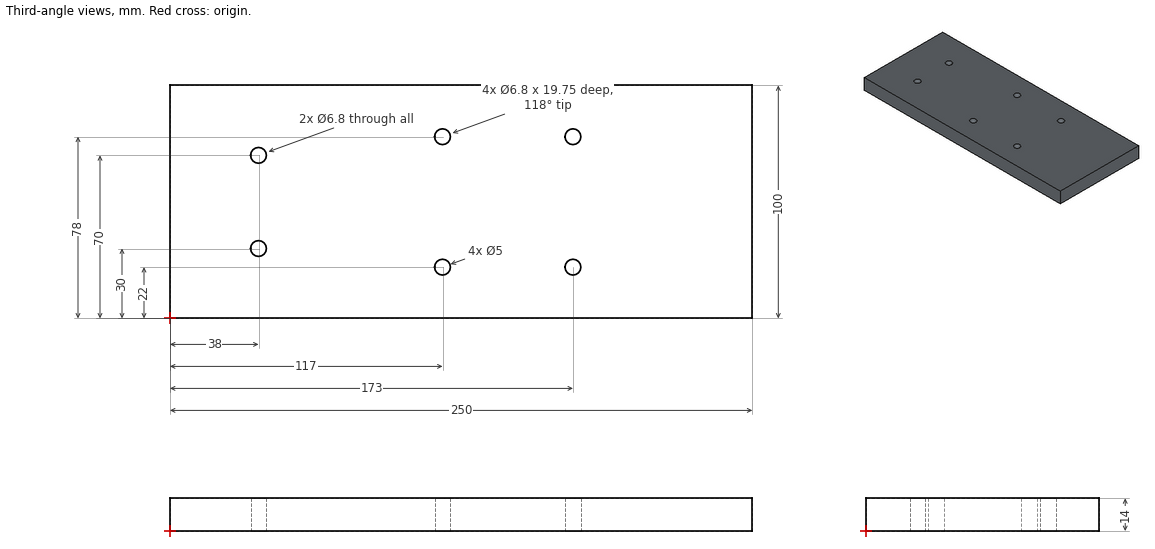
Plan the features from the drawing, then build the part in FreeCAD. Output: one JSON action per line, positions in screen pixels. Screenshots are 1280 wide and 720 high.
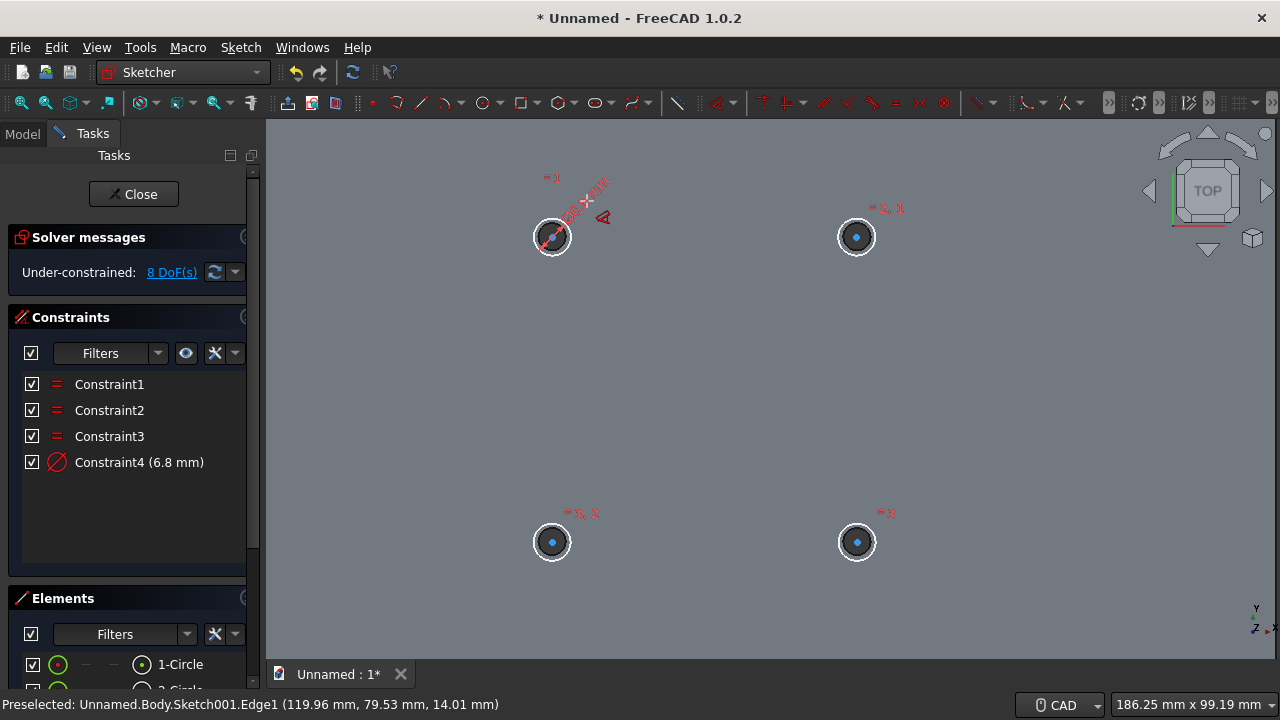
{"action": "left_click", "coordinate": [552, 237]}
{"action": "left_click", "coordinate": [586, 434]}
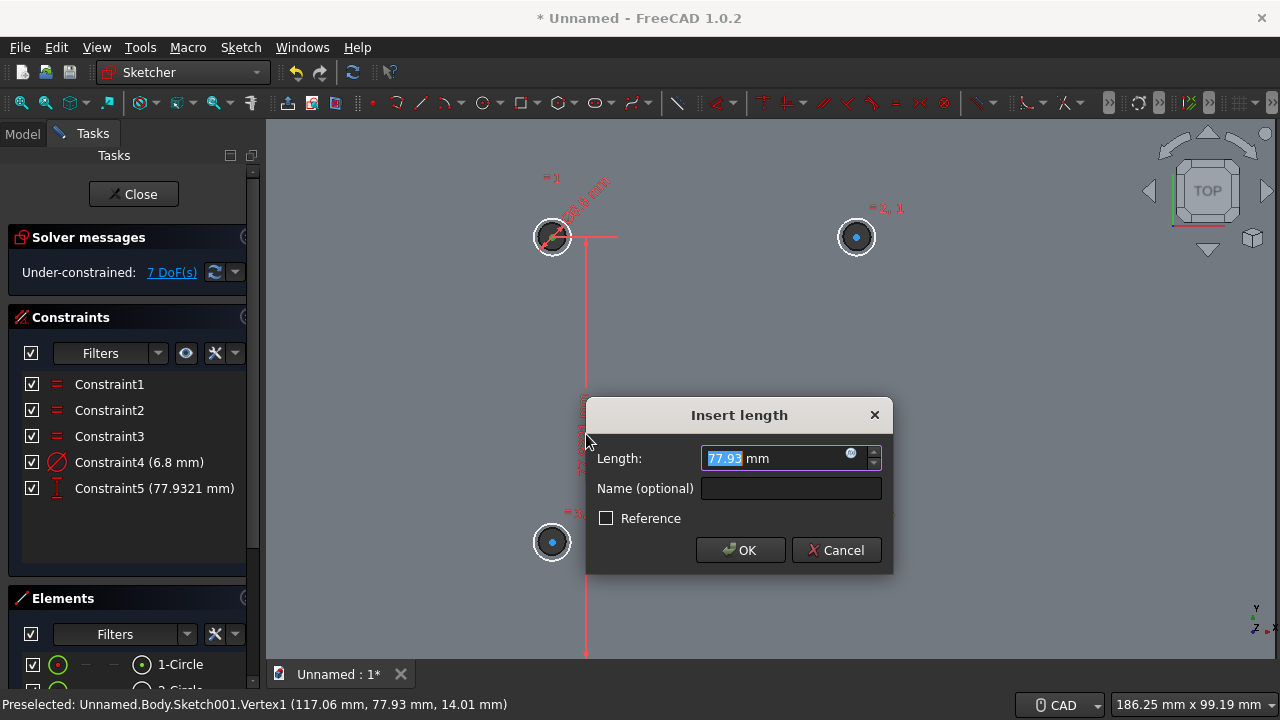
{"action": "type", "text": "78"}
{"action": "key", "text": "Return"}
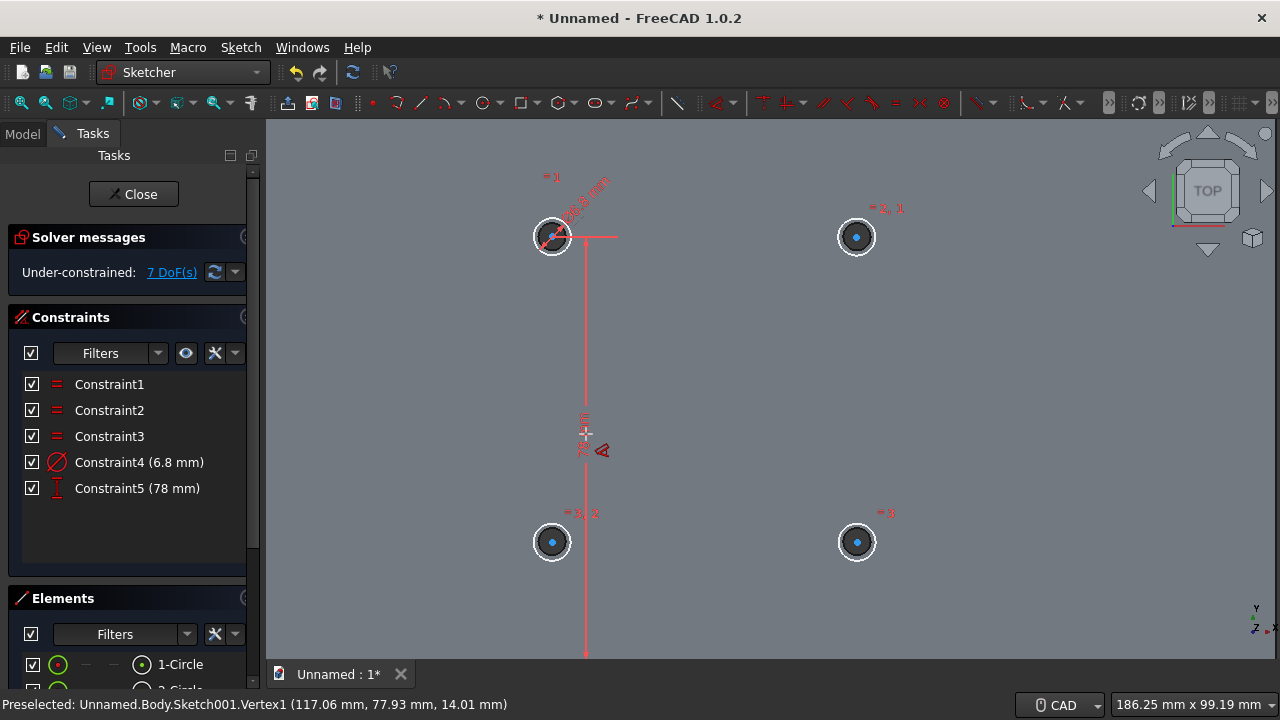
{"action": "left_click", "coordinate": [857, 237]}
{"action": "left_click", "coordinate": [891, 434]}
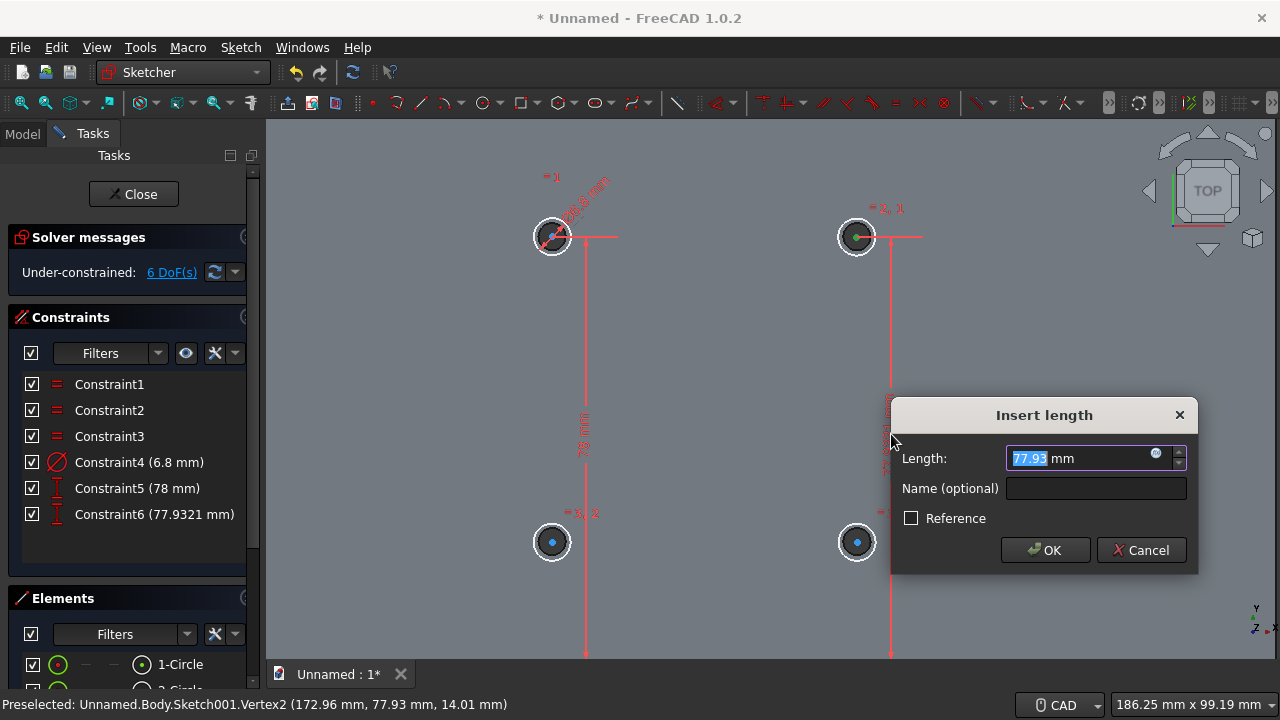
{"action": "type", "text": "78"}
{"action": "key", "text": "Return"}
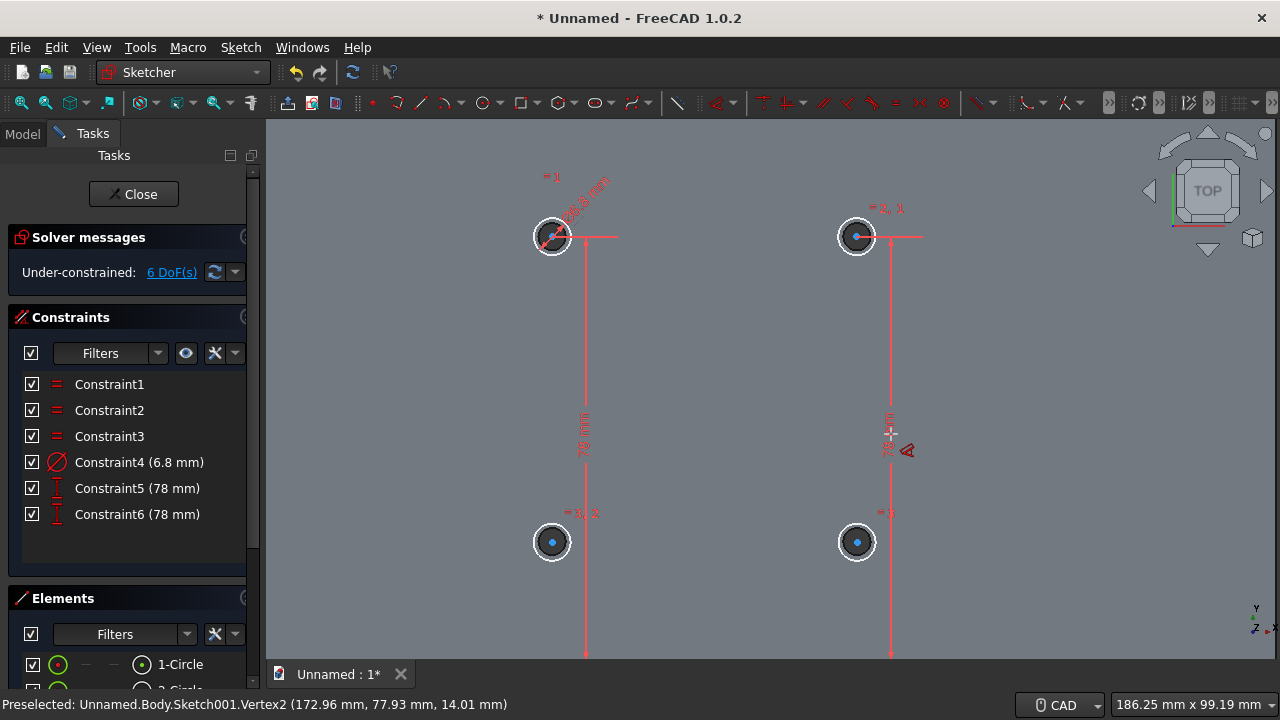
{"action": "left_click", "coordinate": [552, 542]}
{"action": "left_click", "coordinate": [586, 587]}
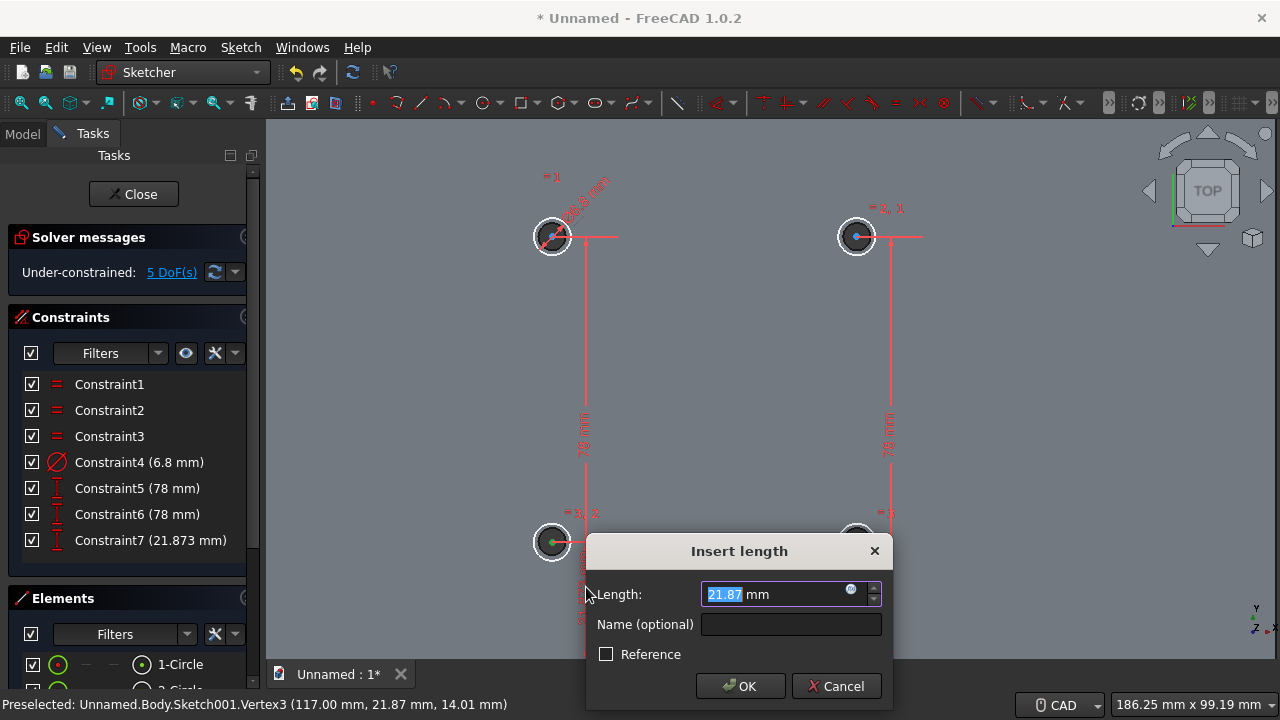
{"action": "type", "text": "22"}
{"action": "key", "text": "Return"}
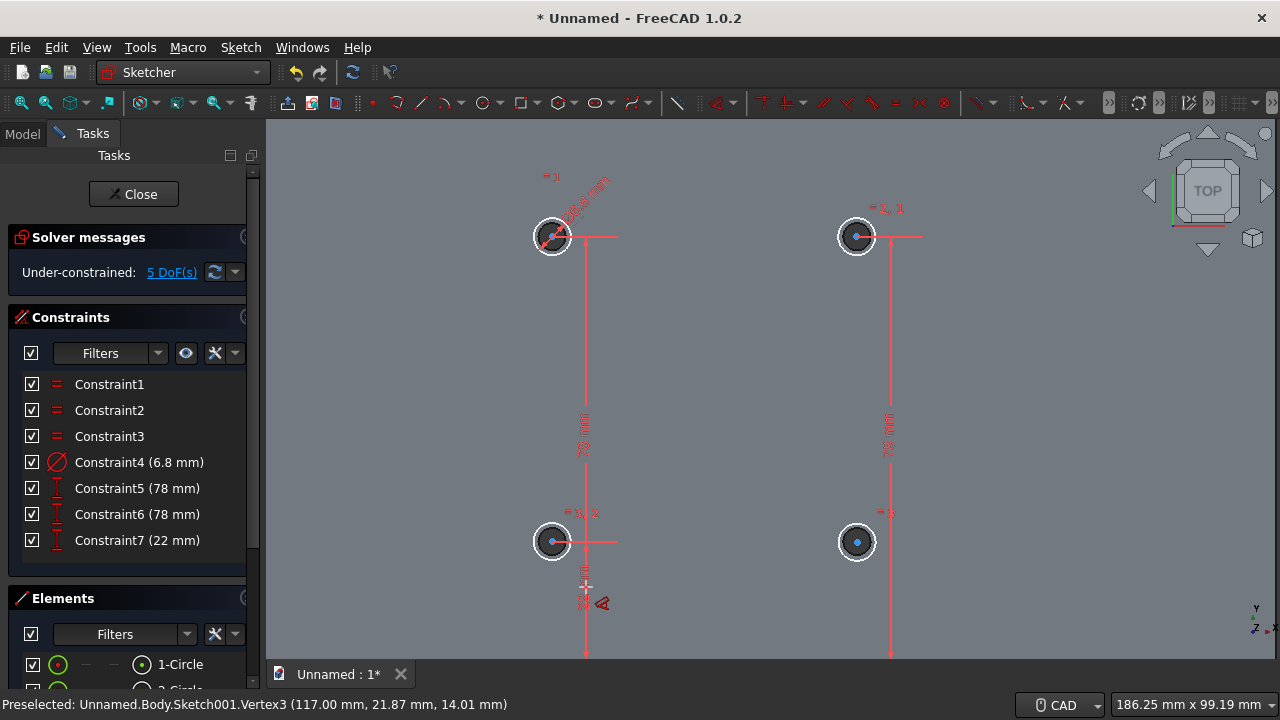
{"action": "left_click", "coordinate": [857, 542]}
{"action": "left_click", "coordinate": [891, 587]}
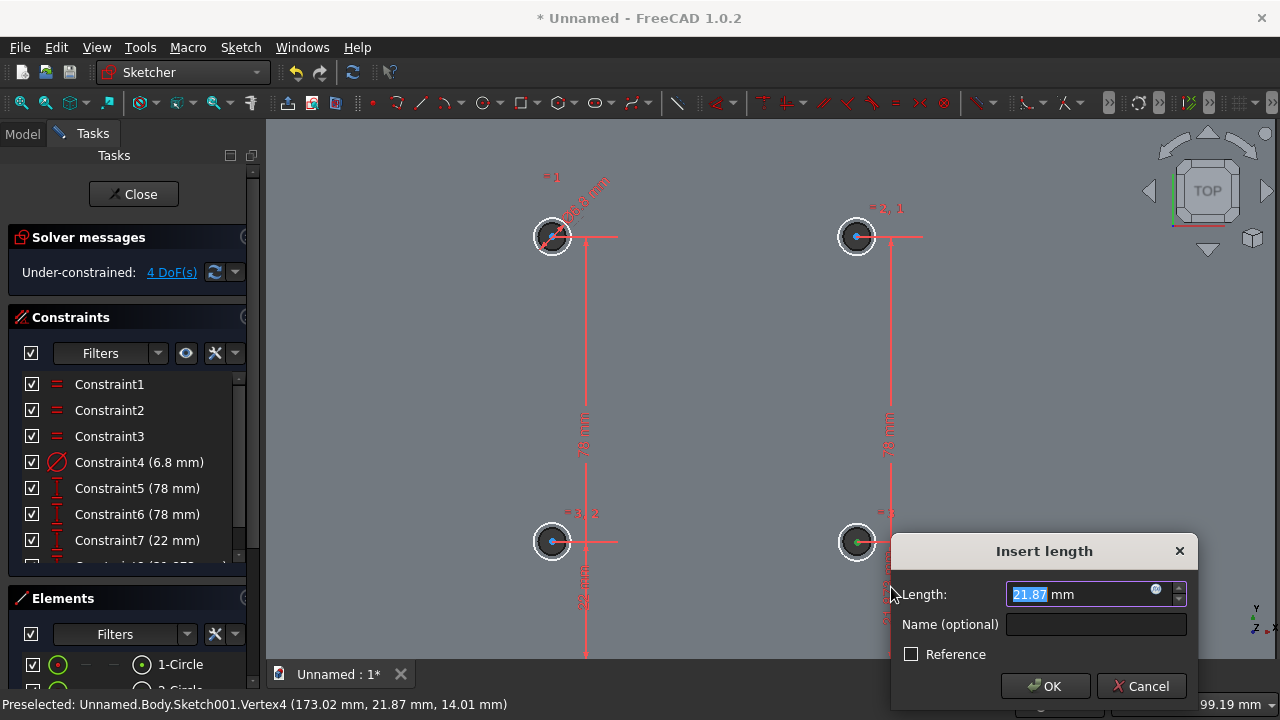
{"action": "type", "text": "22"}
{"action": "key", "text": "Return"}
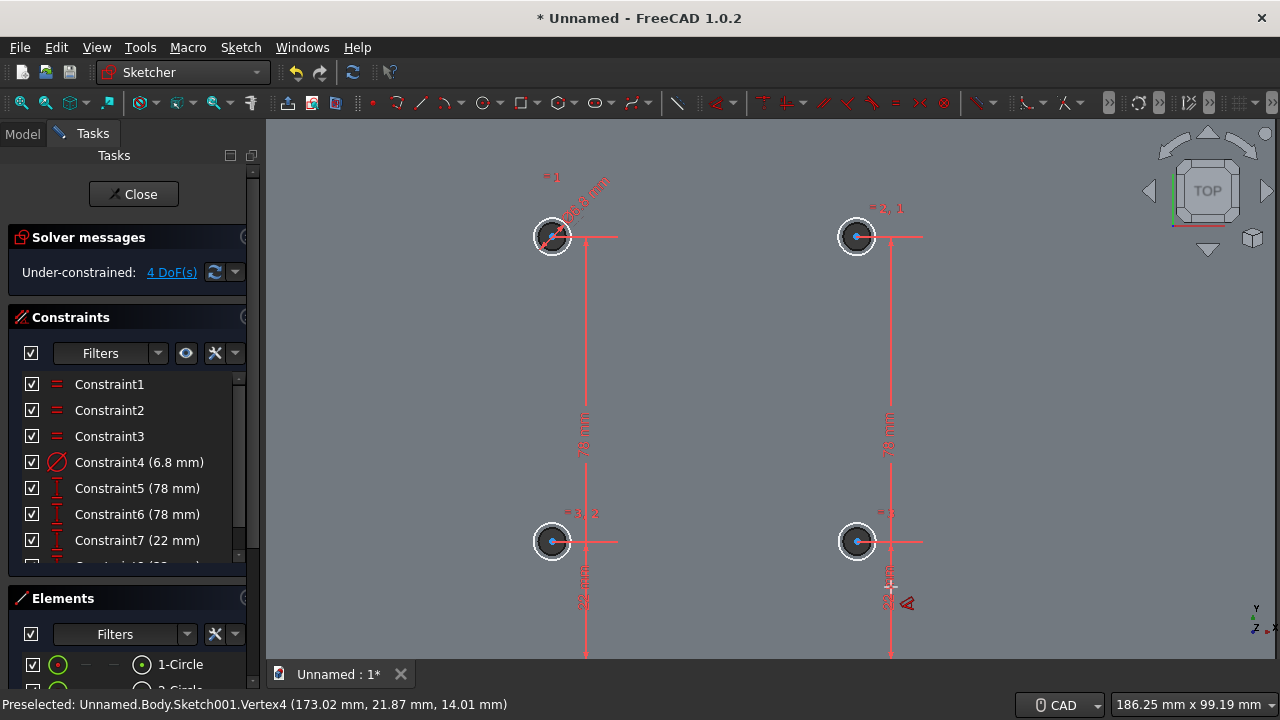
{"action": "left_click", "coordinate": [552, 237]}
{"action": "left_click", "coordinate": [423, 203]}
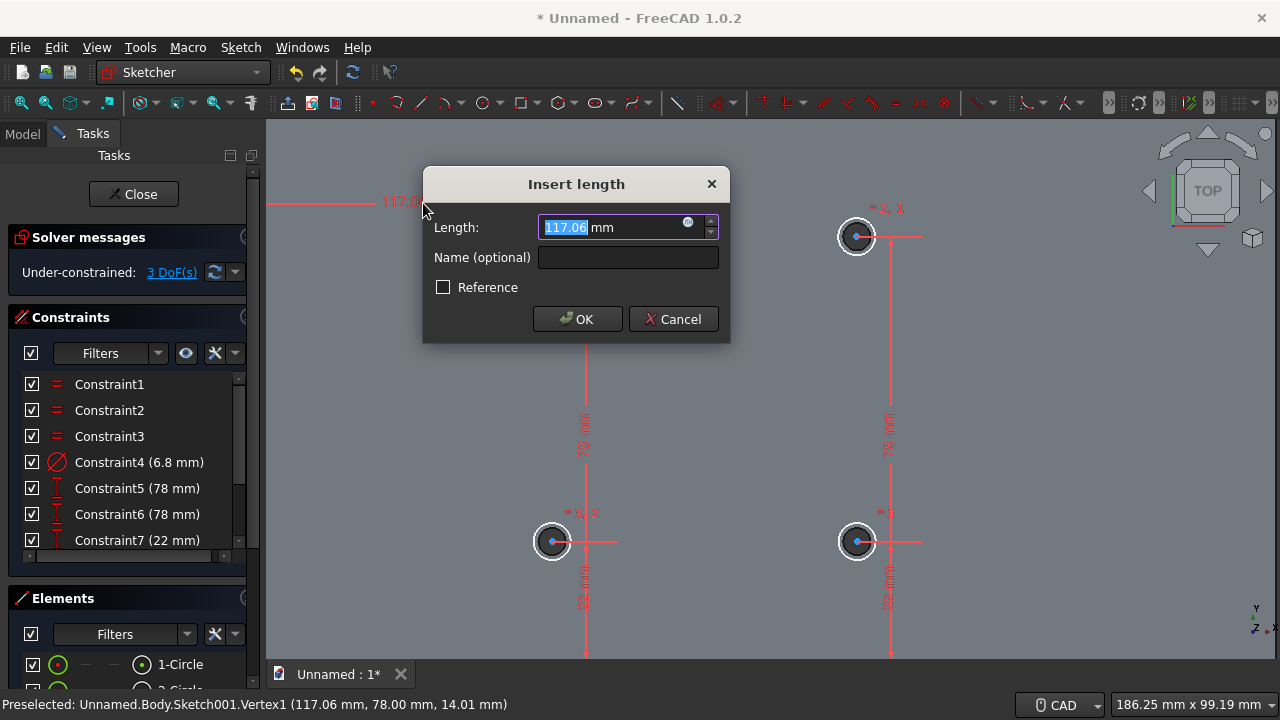
{"action": "type", "text": "117"}
{"action": "key", "text": "Return"}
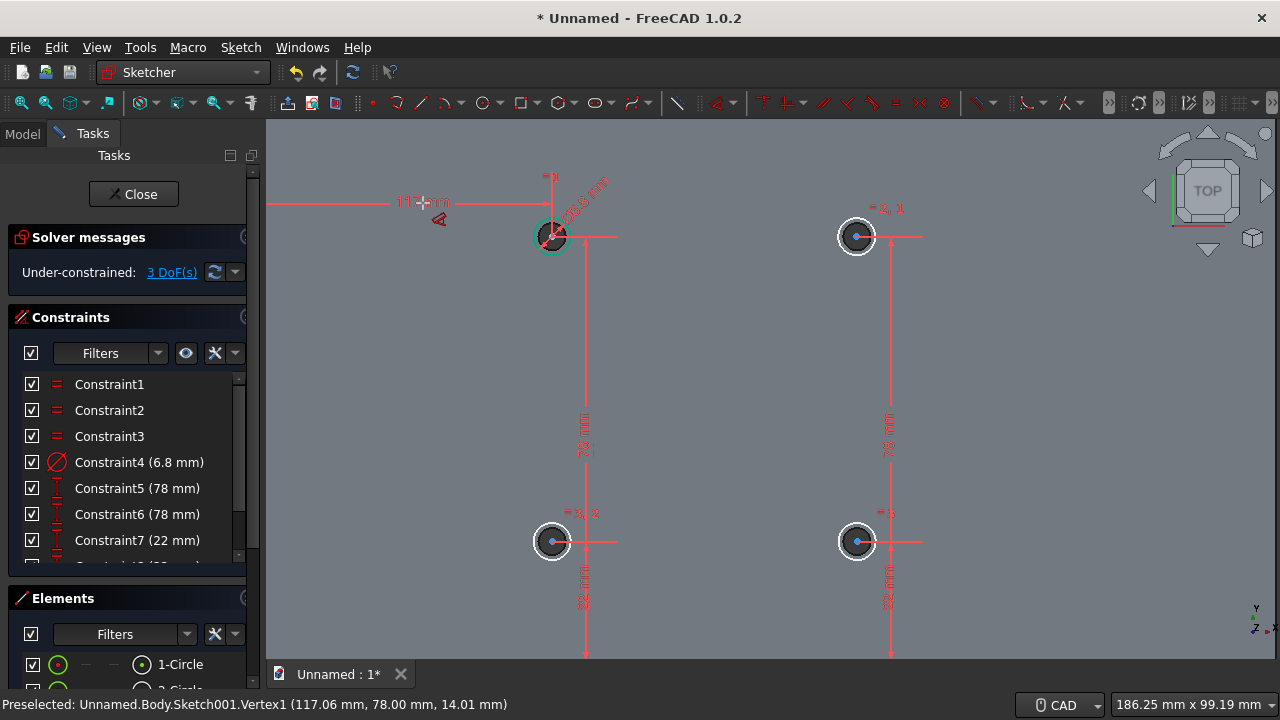
{"action": "left_click", "coordinate": [857, 237]}
{"action": "left_click", "coordinate": [705, 203]}